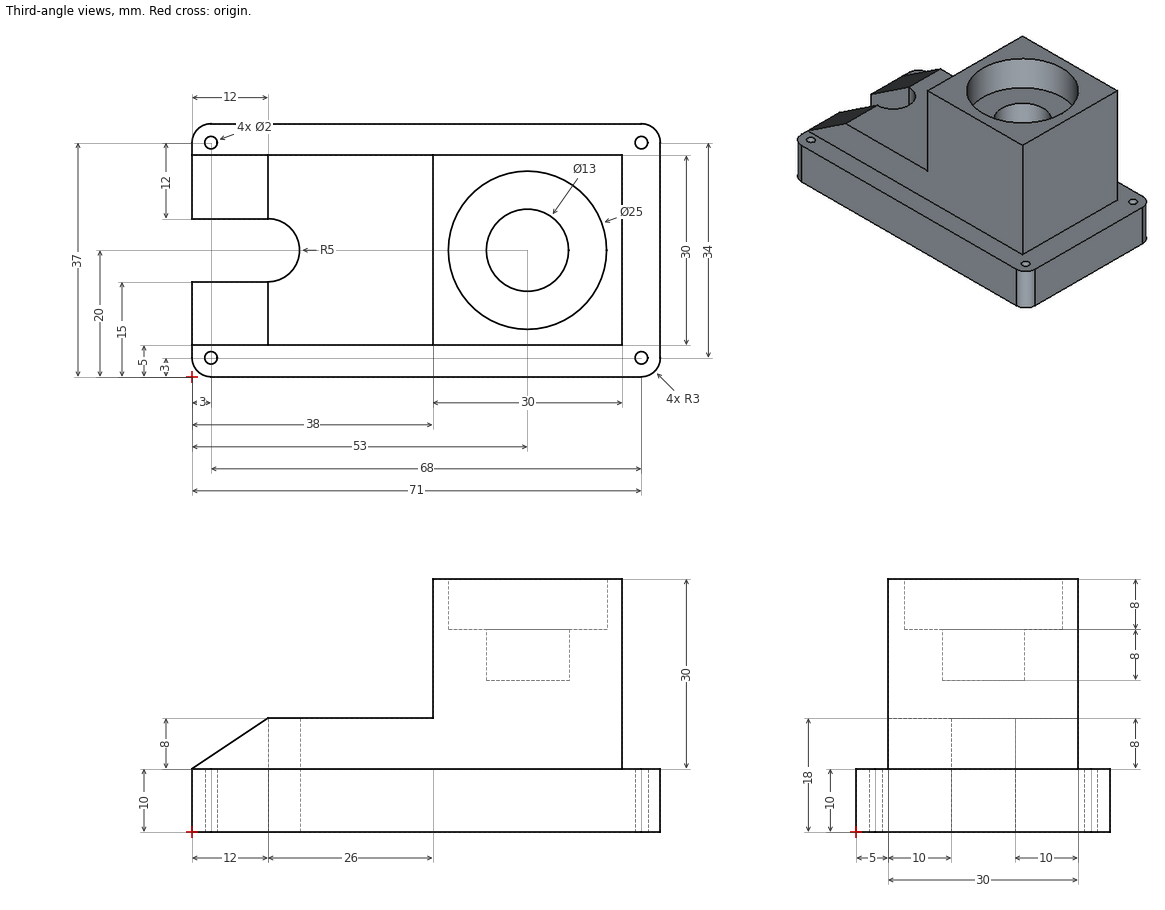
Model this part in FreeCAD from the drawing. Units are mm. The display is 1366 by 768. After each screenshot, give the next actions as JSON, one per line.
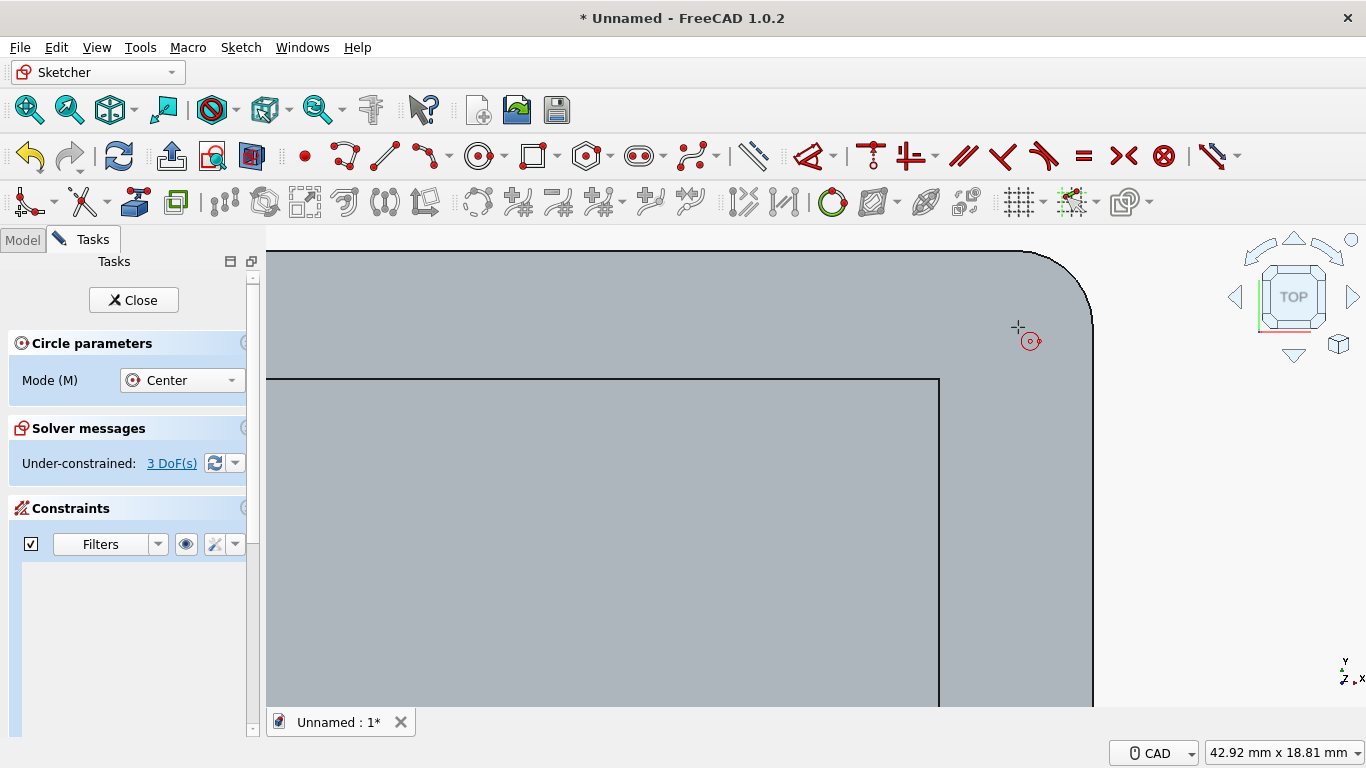
{"action": "left_click", "coordinate": [1016, 328]}
{"action": "left_click", "coordinate": [1034, 309]}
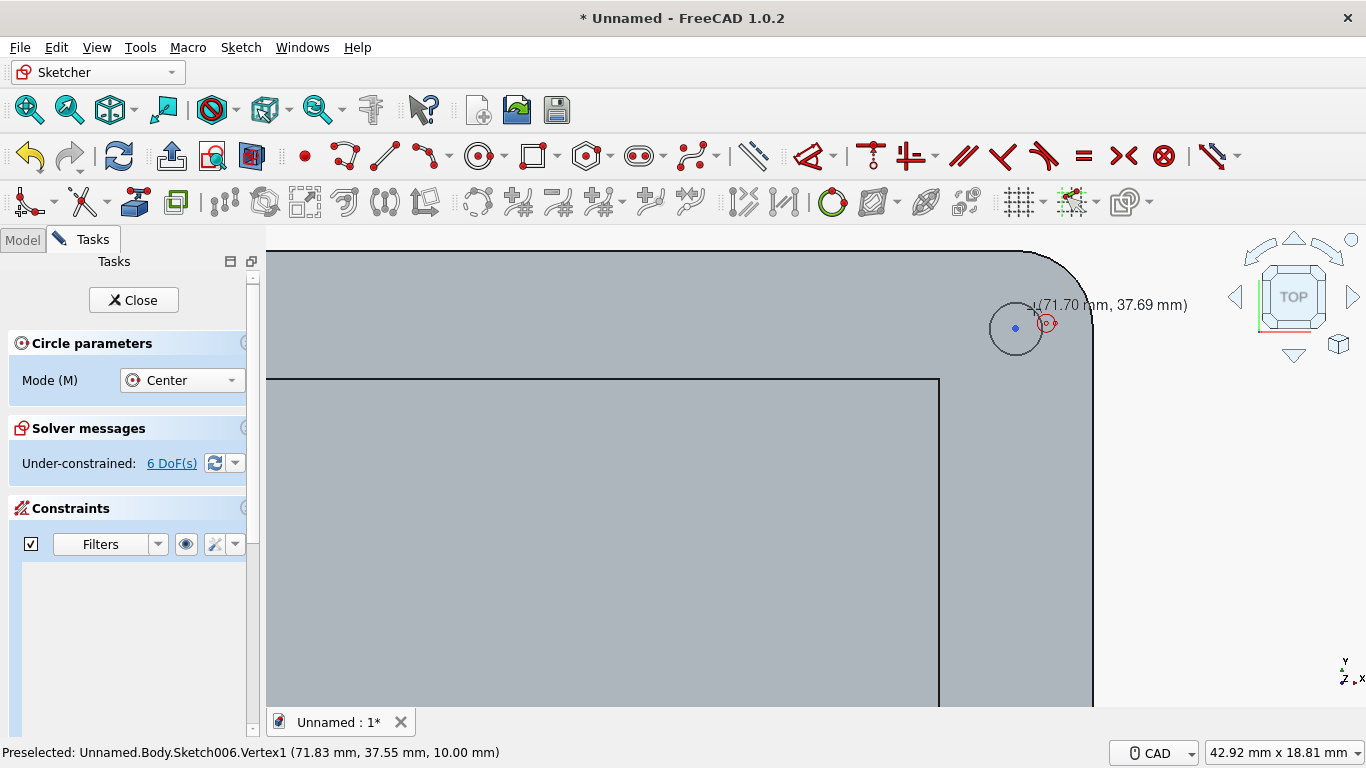
{"action": "scroll", "coordinate": [1018, 327], "scroll_direction": "down", "scroll_amount": 6}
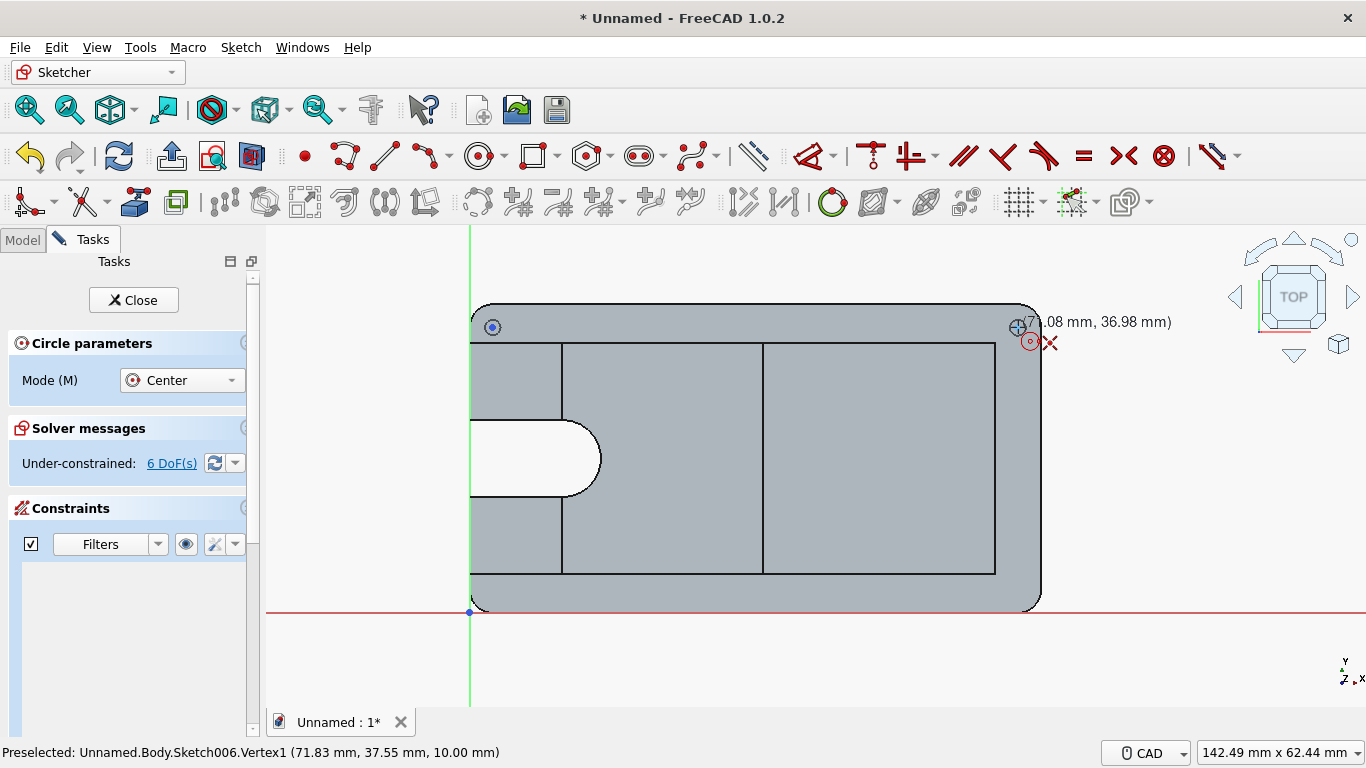
{"action": "scroll", "coordinate": [1018, 590], "scroll_direction": "up", "scroll_amount": 6}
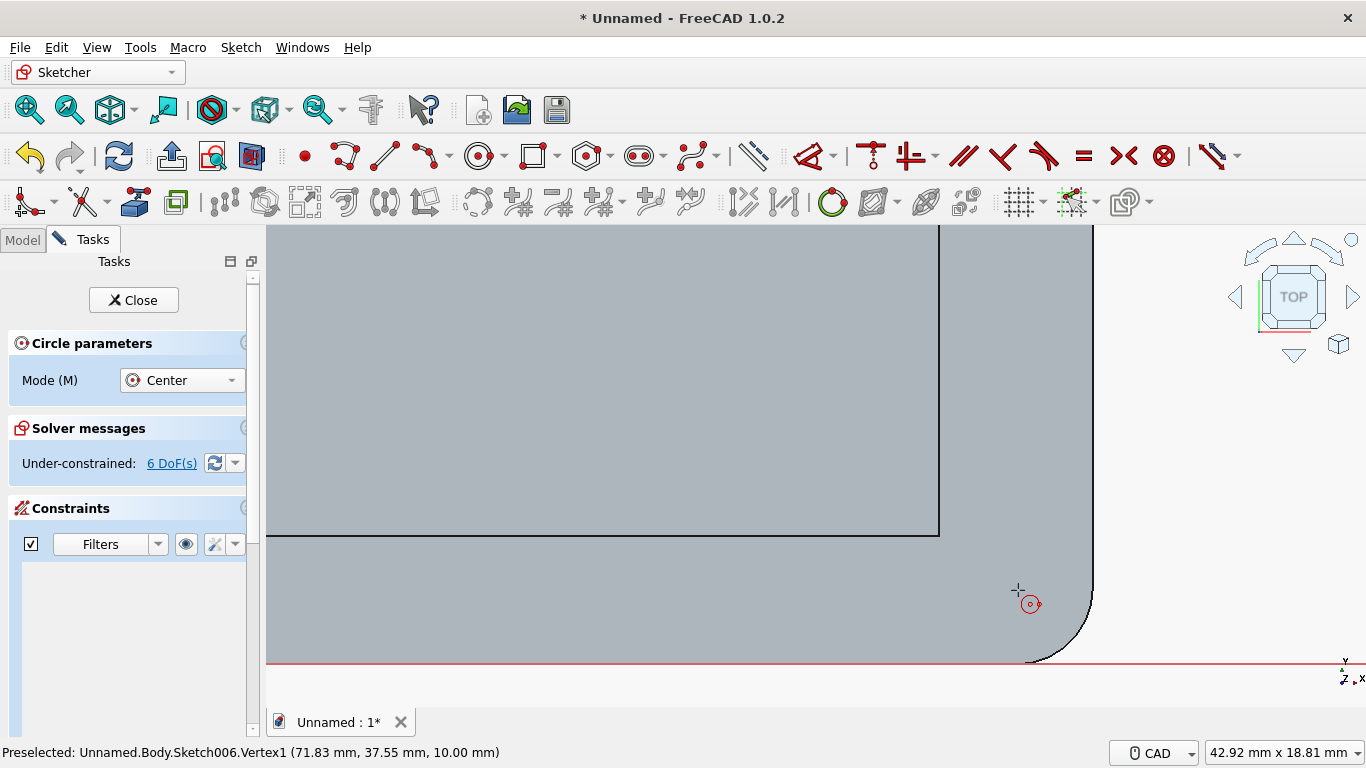
{"action": "left_click", "coordinate": [1016, 588]}
{"action": "left_click", "coordinate": [1034, 569]}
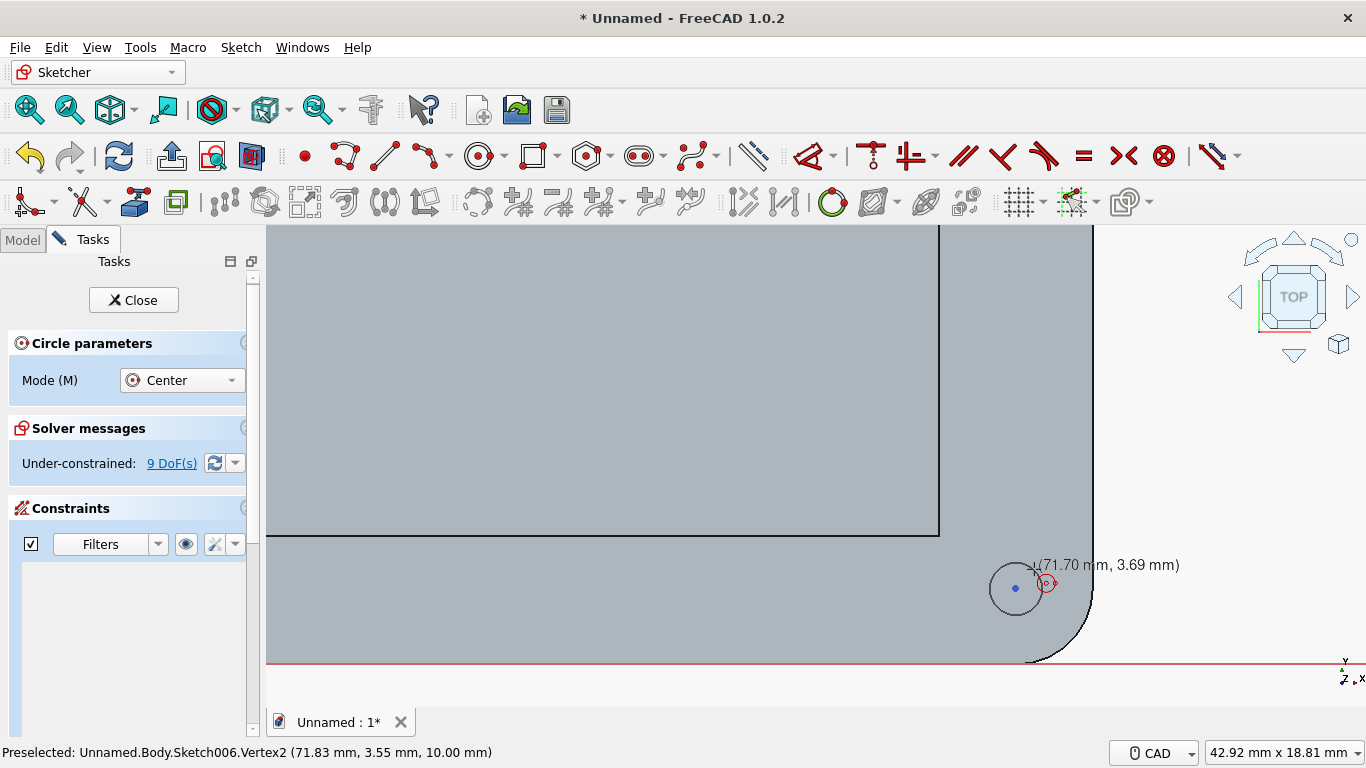
{"action": "scroll", "coordinate": [1018, 590], "scroll_direction": "down", "scroll_amount": 6}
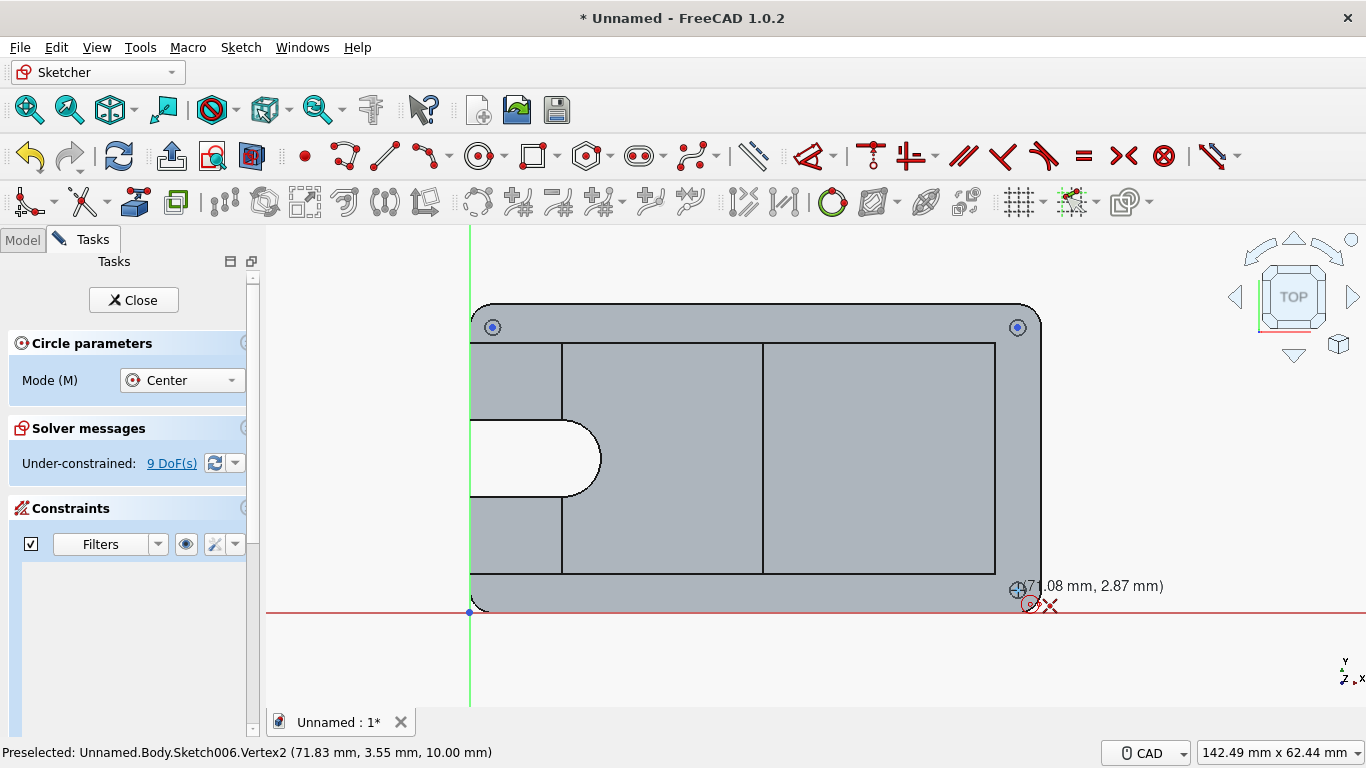
{"action": "scroll", "coordinate": [493, 590], "scroll_direction": "up", "scroll_amount": 6}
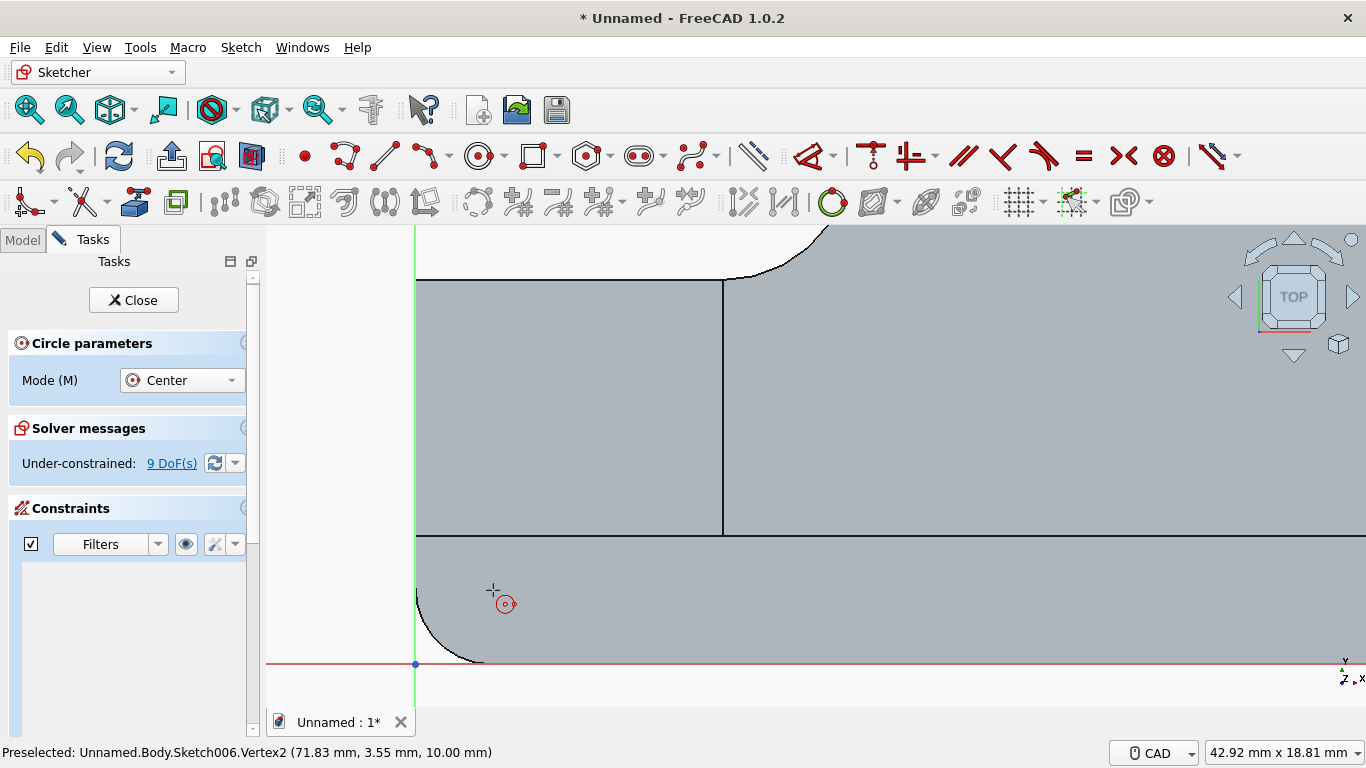
{"action": "left_click", "coordinate": [492, 588]}
{"action": "left_click", "coordinate": [510, 569]}
{"action": "key", "text": "Escape"}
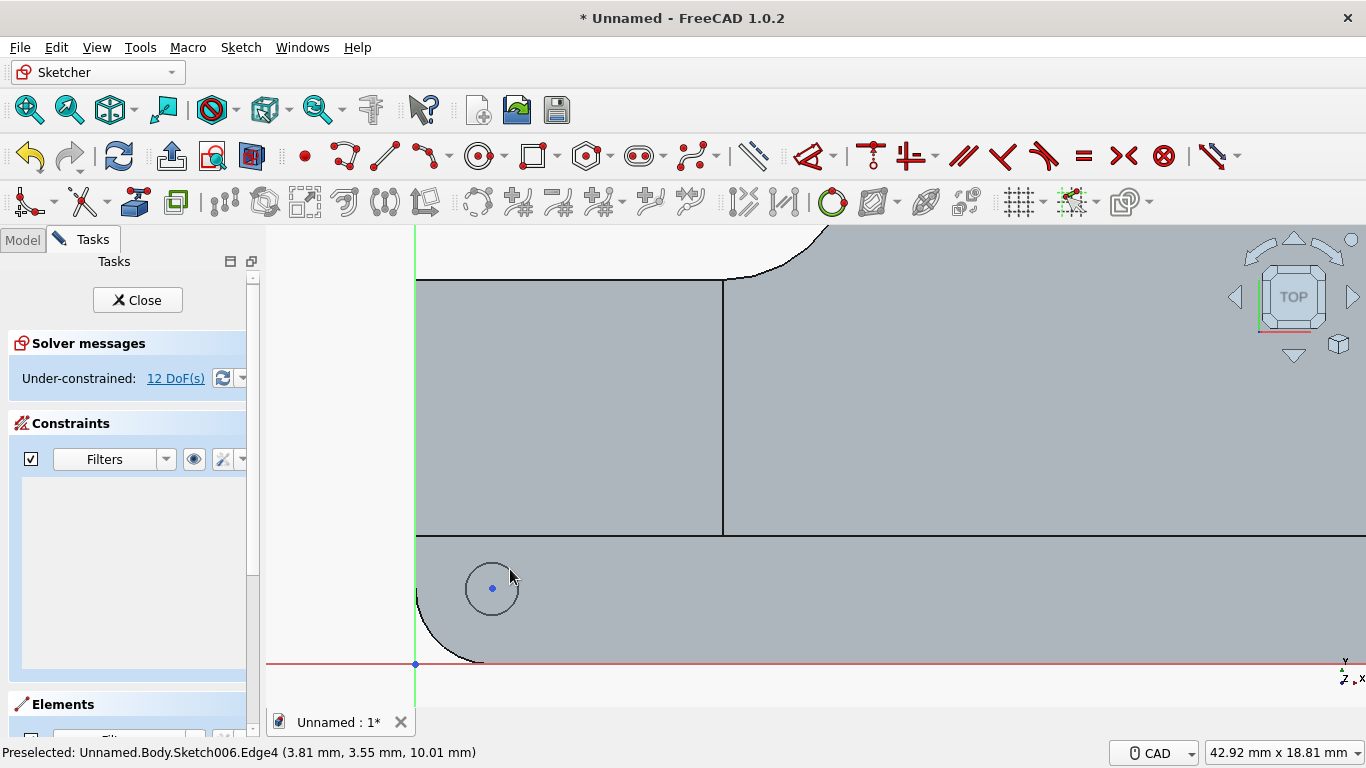
{"action": "scroll", "coordinate": [493, 590], "scroll_direction": "down", "scroll_amount": 6}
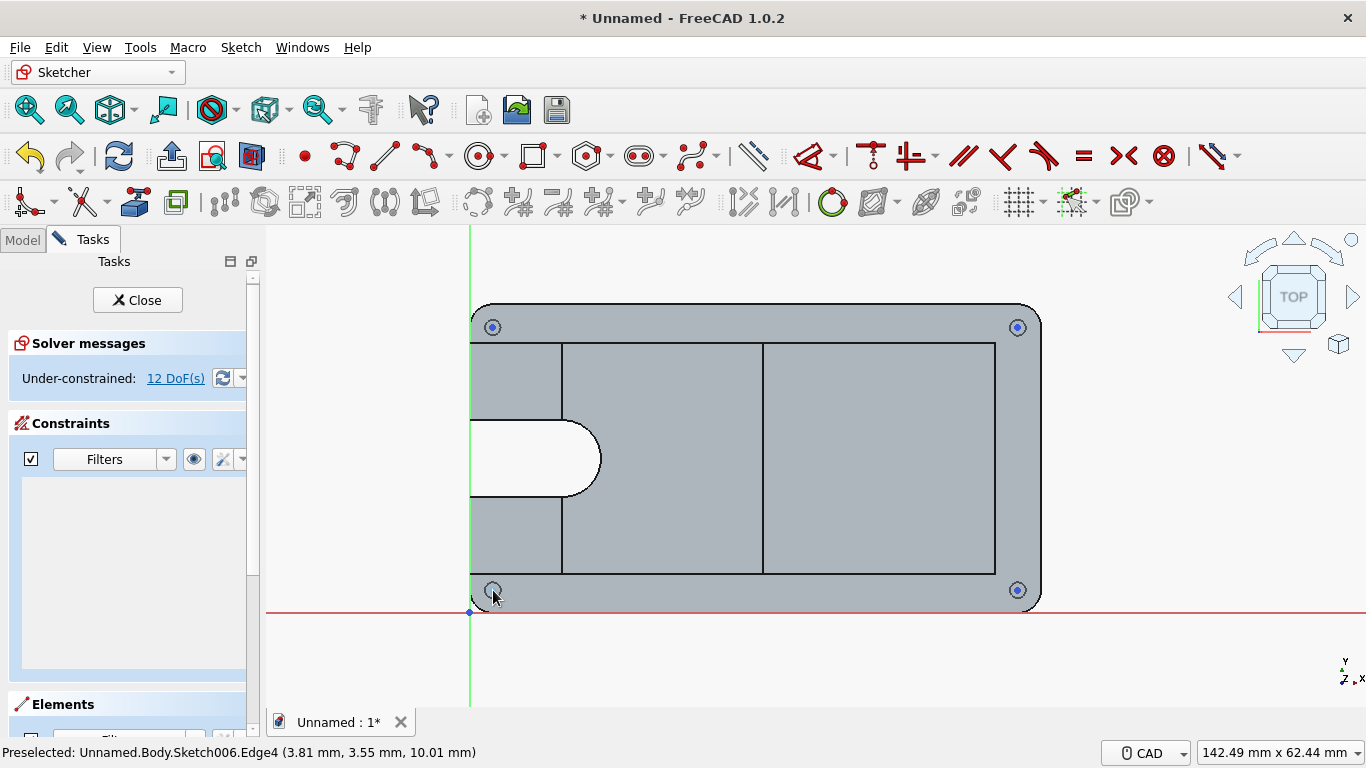
{"action": "scroll", "coordinate": [498, 322], "scroll_direction": "up", "scroll_amount": 3}